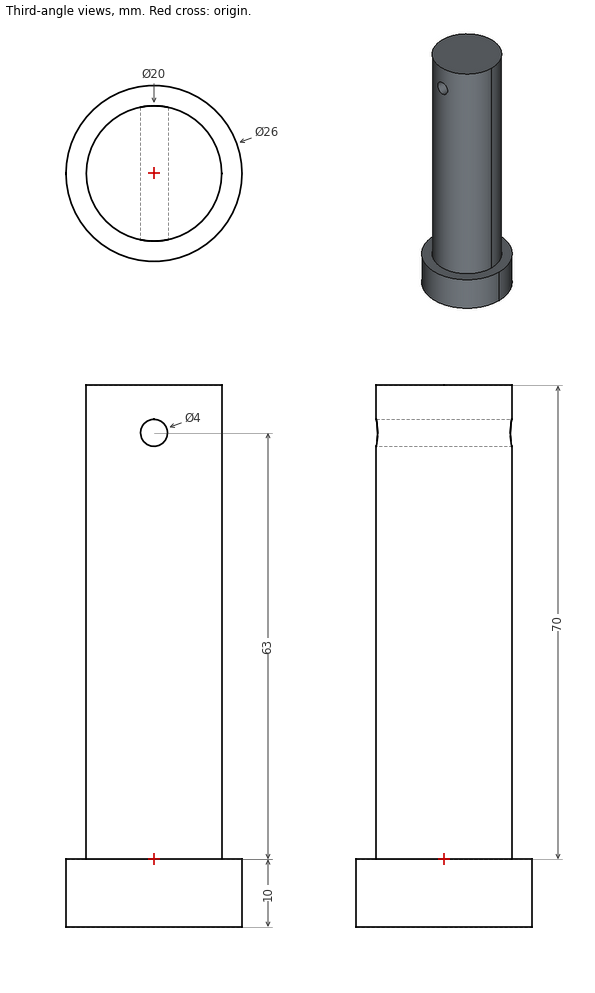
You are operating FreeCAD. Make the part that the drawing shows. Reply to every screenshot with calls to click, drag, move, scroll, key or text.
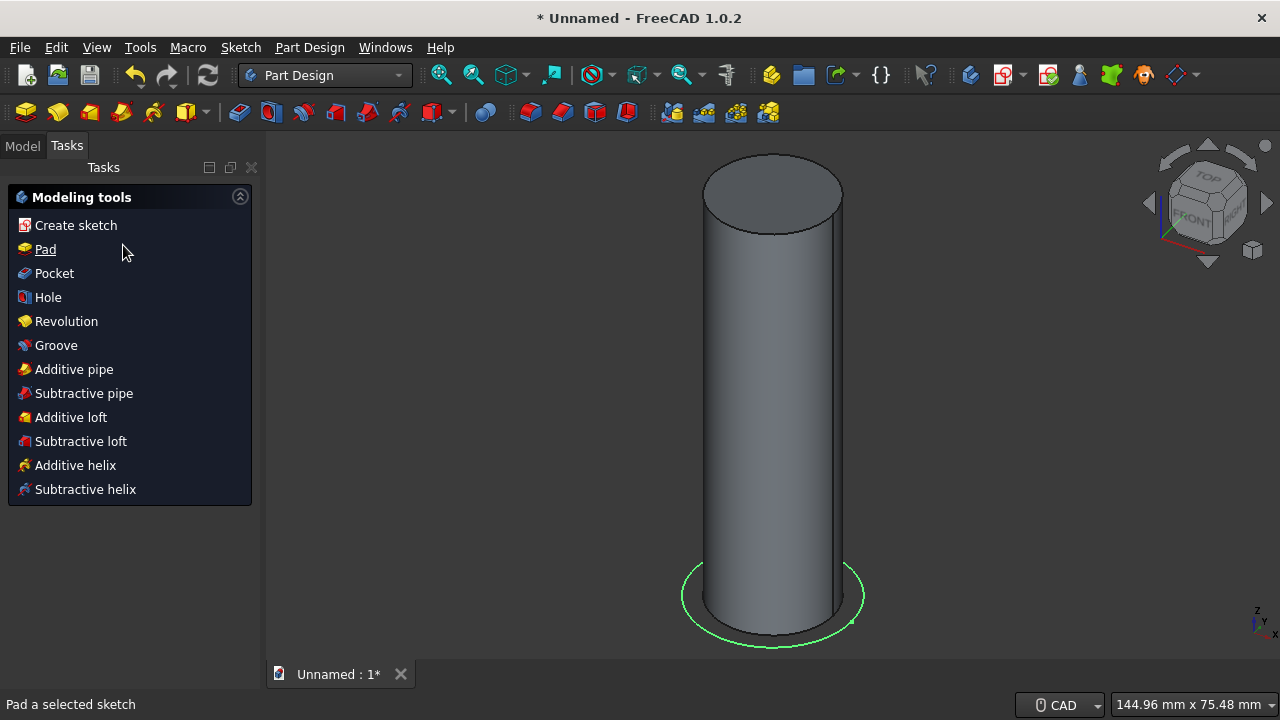
click(26, 112)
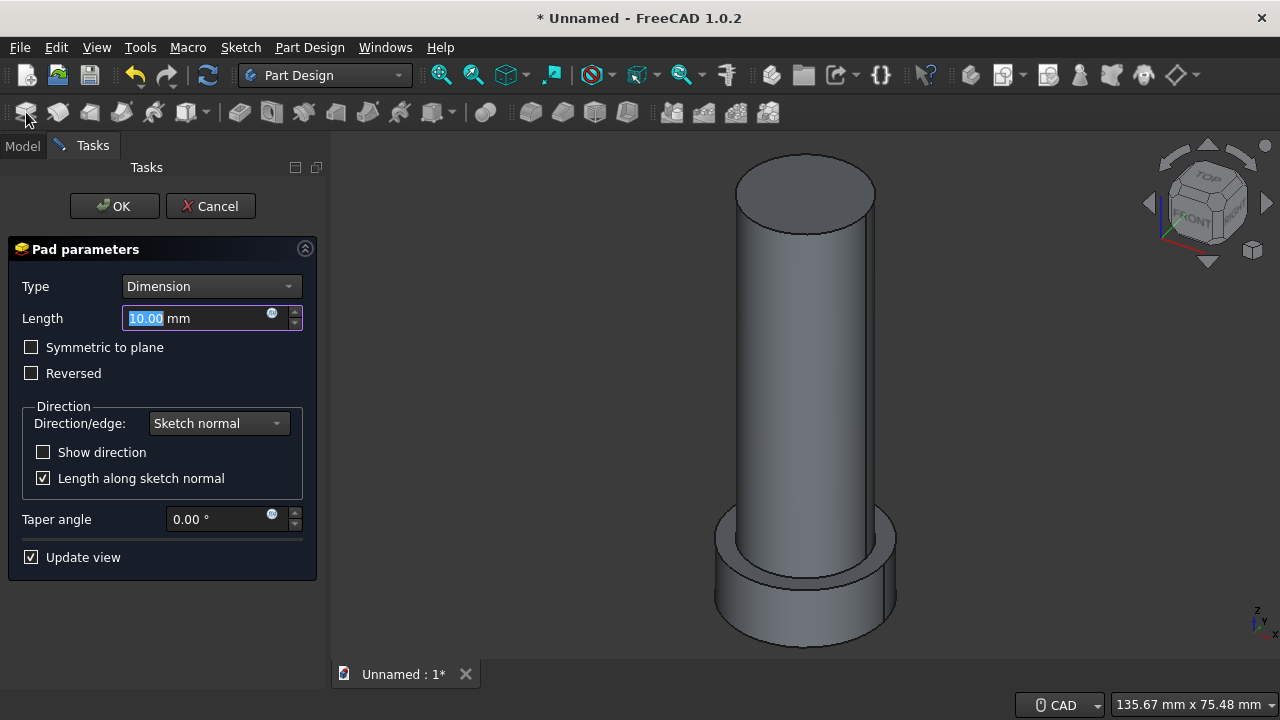
text(10)
key(Tab)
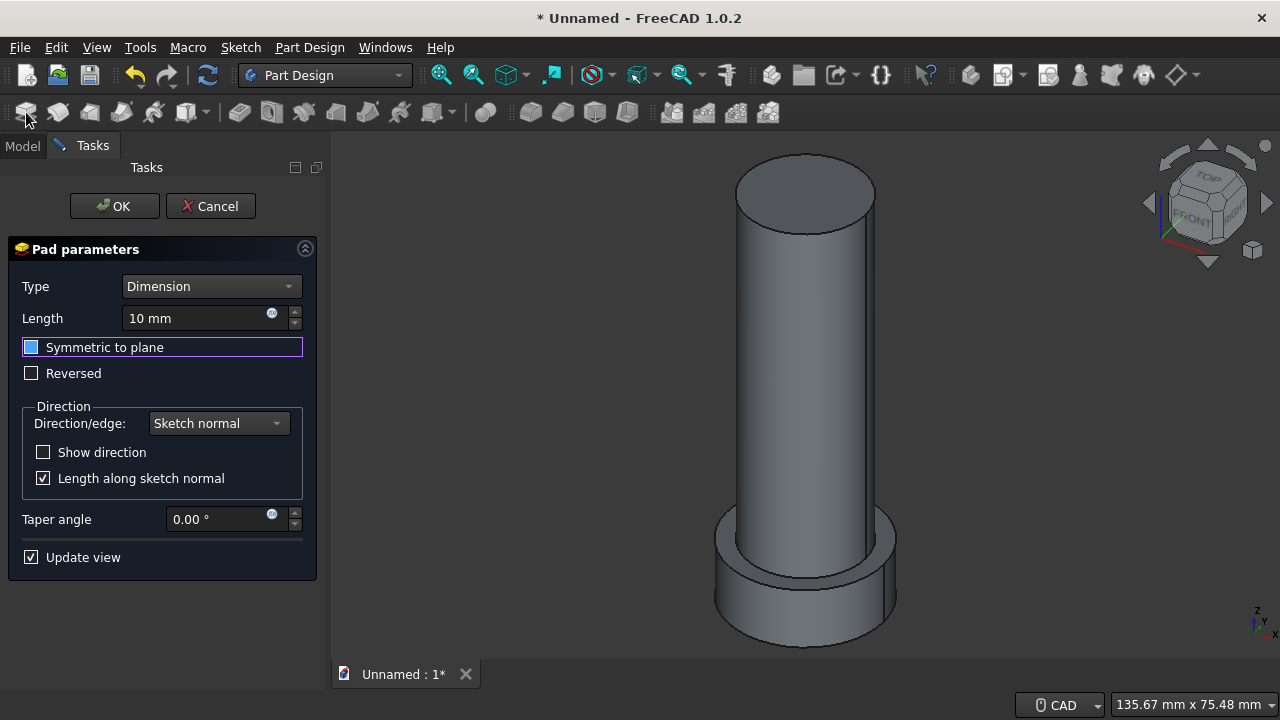
click(30, 373)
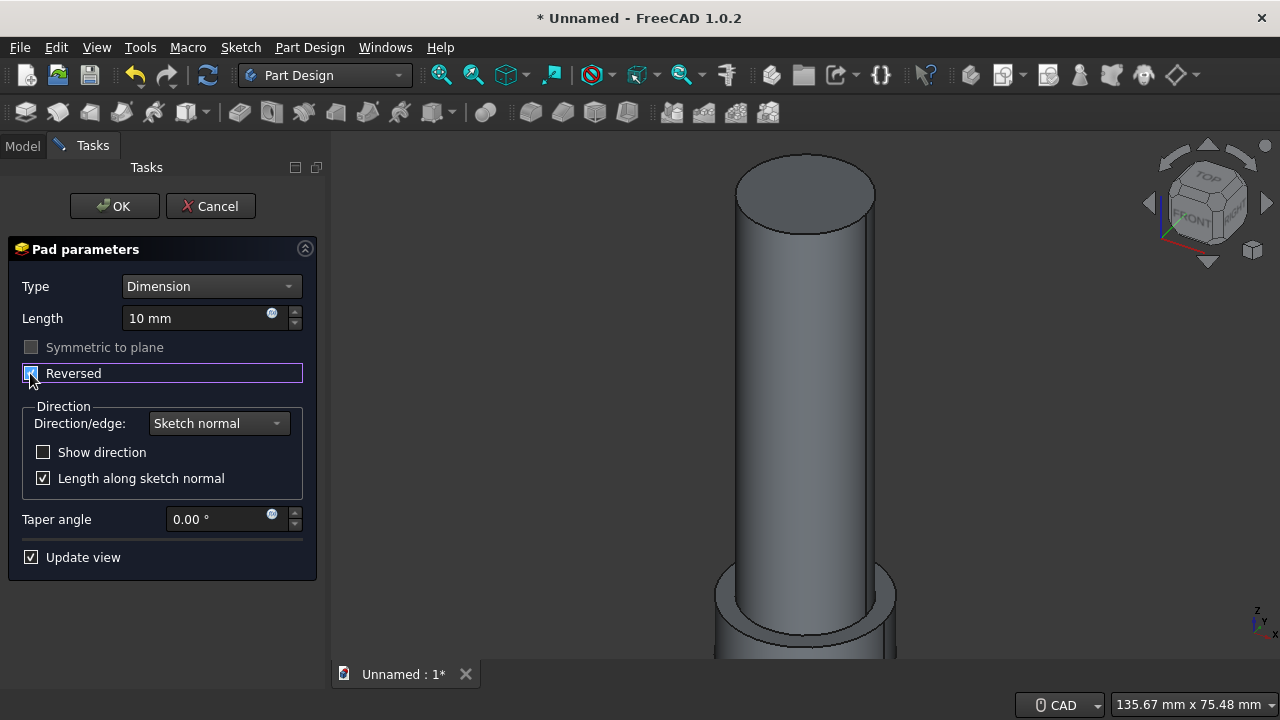
click(115, 206)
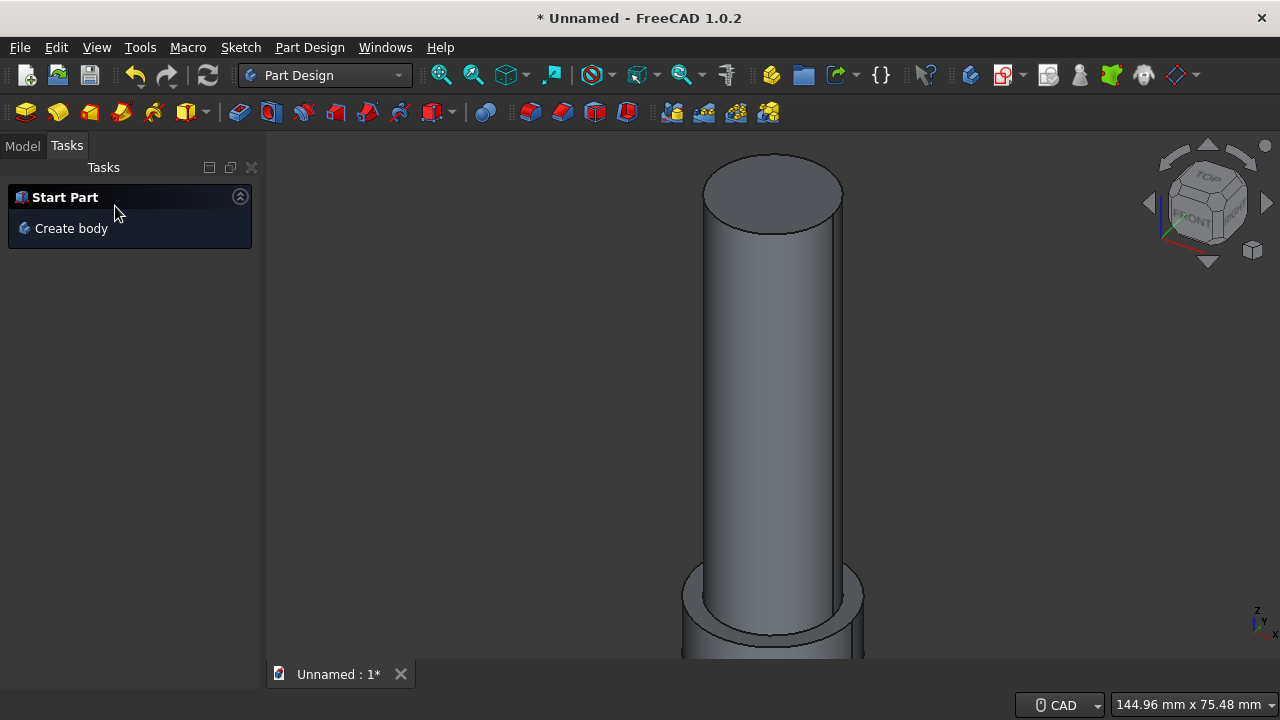
click(442, 76)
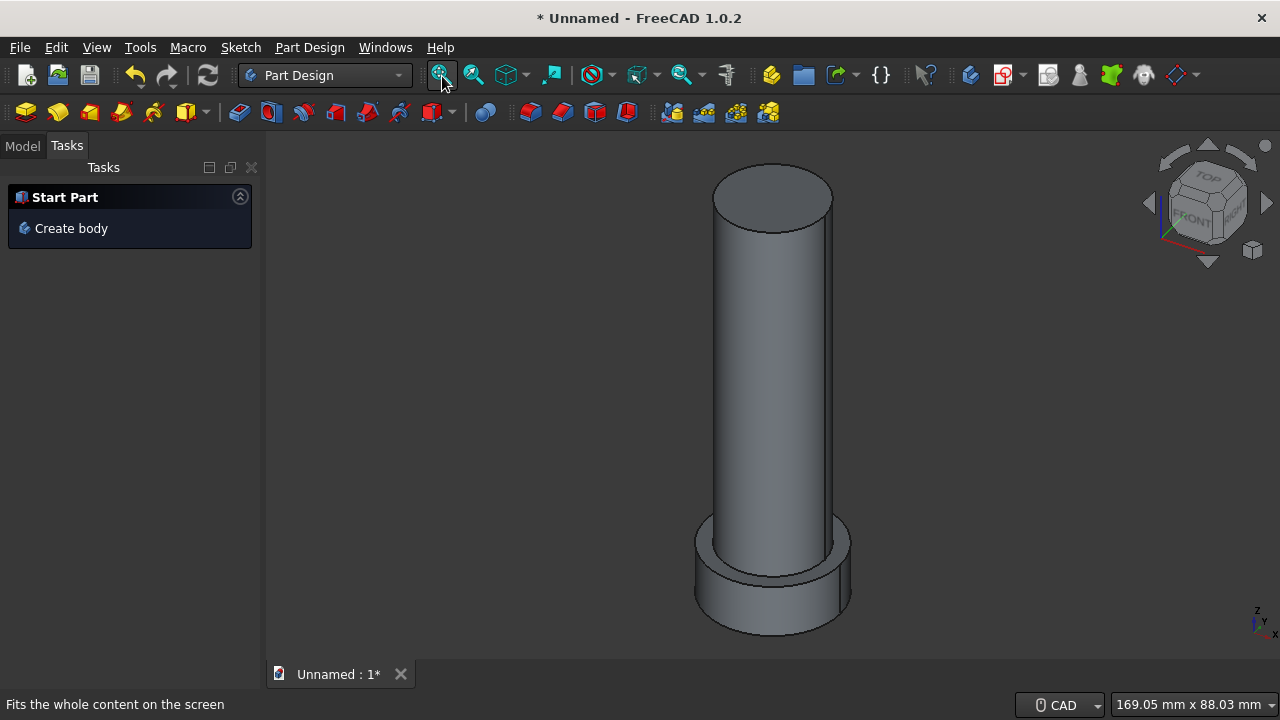
click(1004, 76)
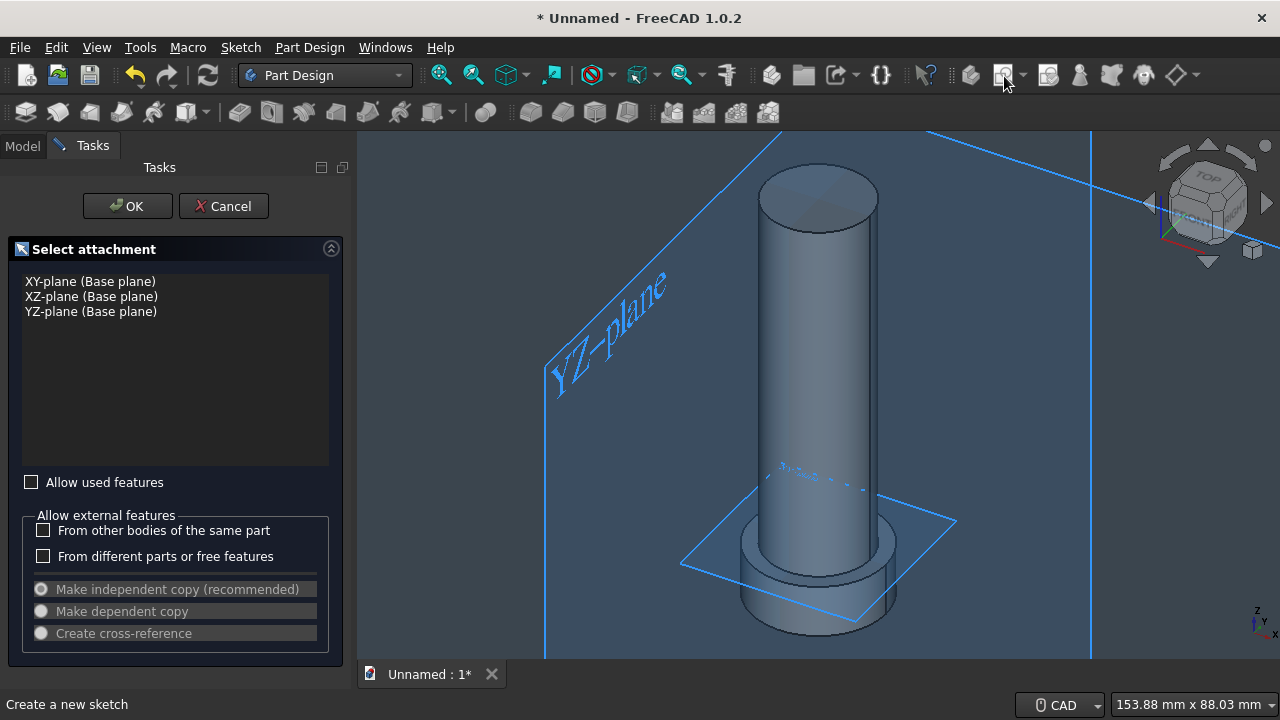
click(82, 296)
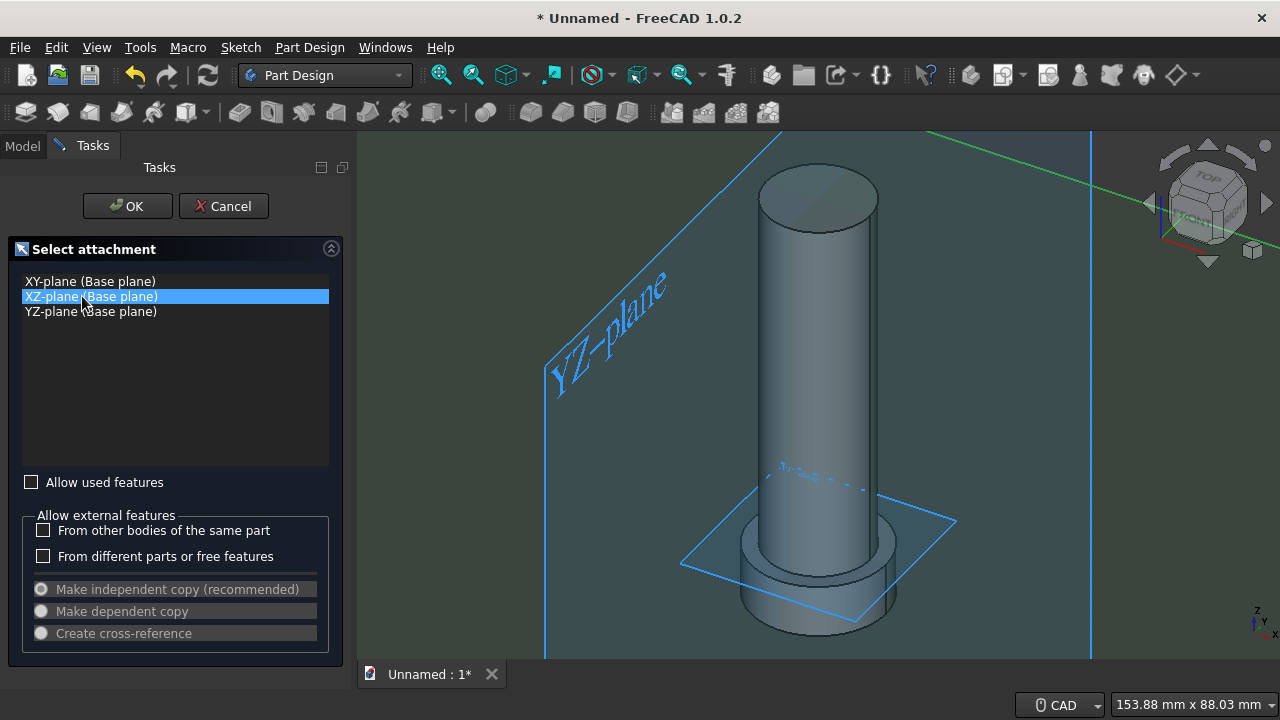
click(128, 206)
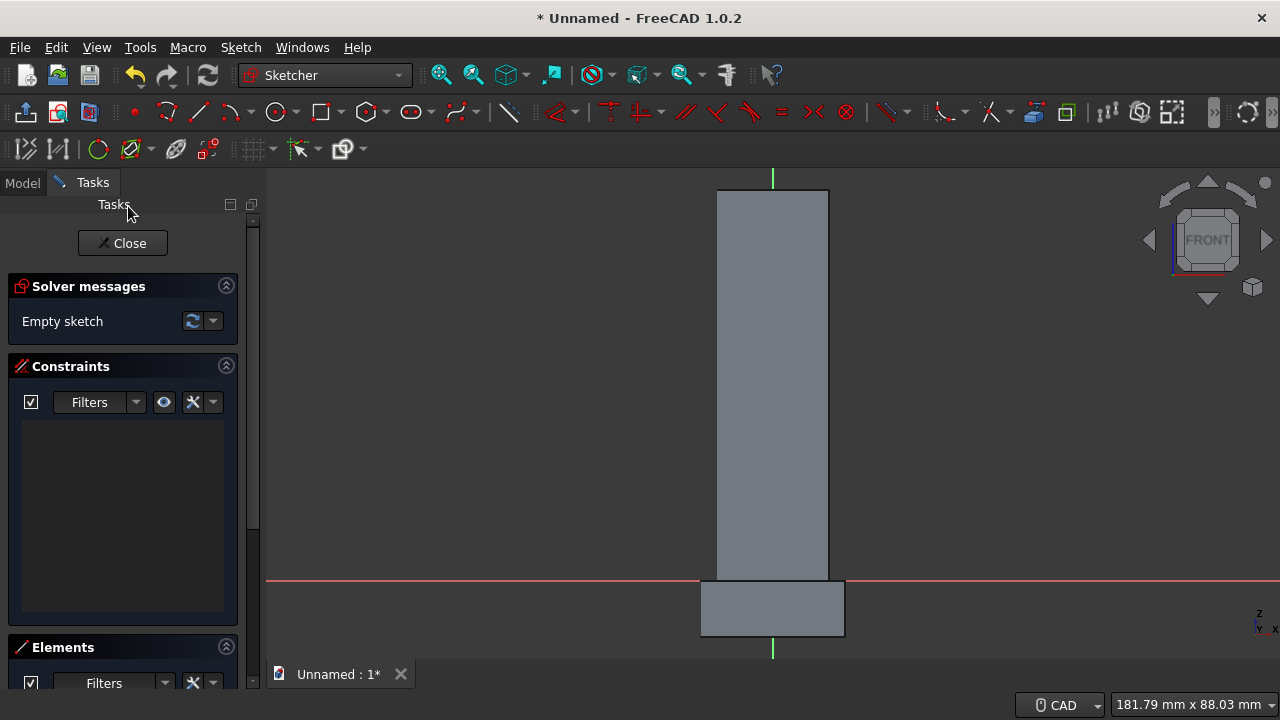
click(90, 112)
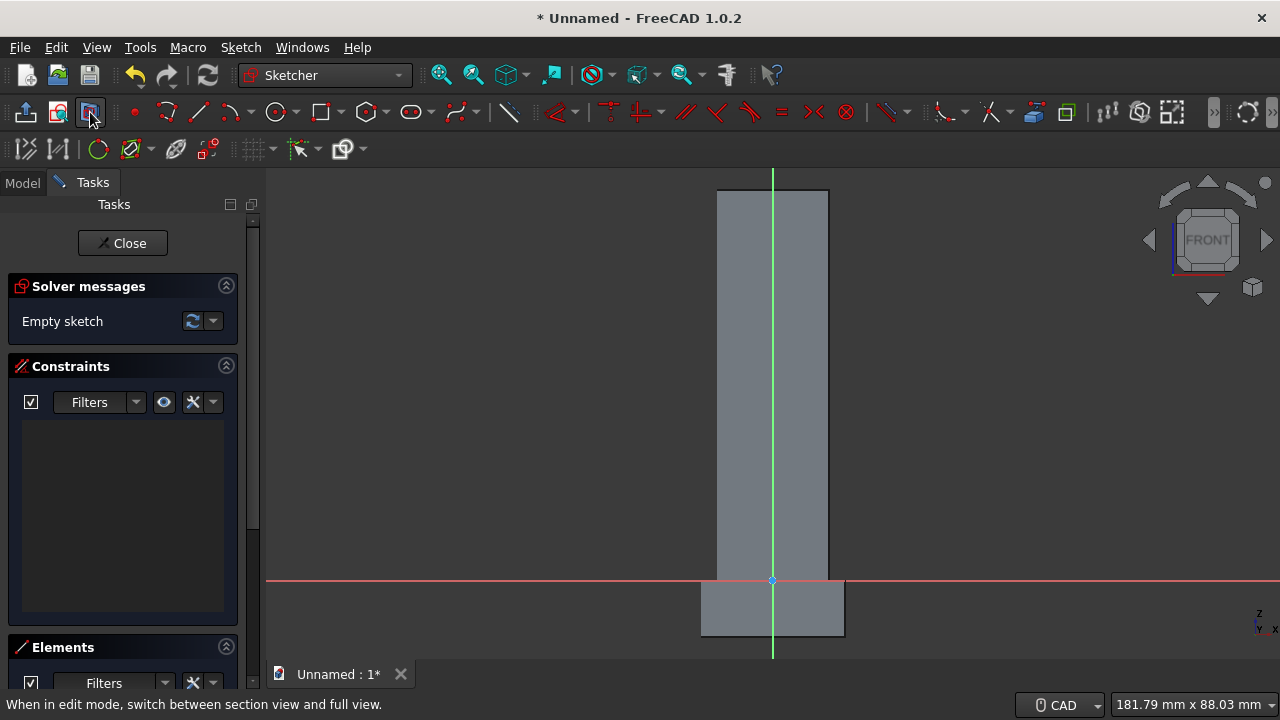
scroll(778, 215, up, 13)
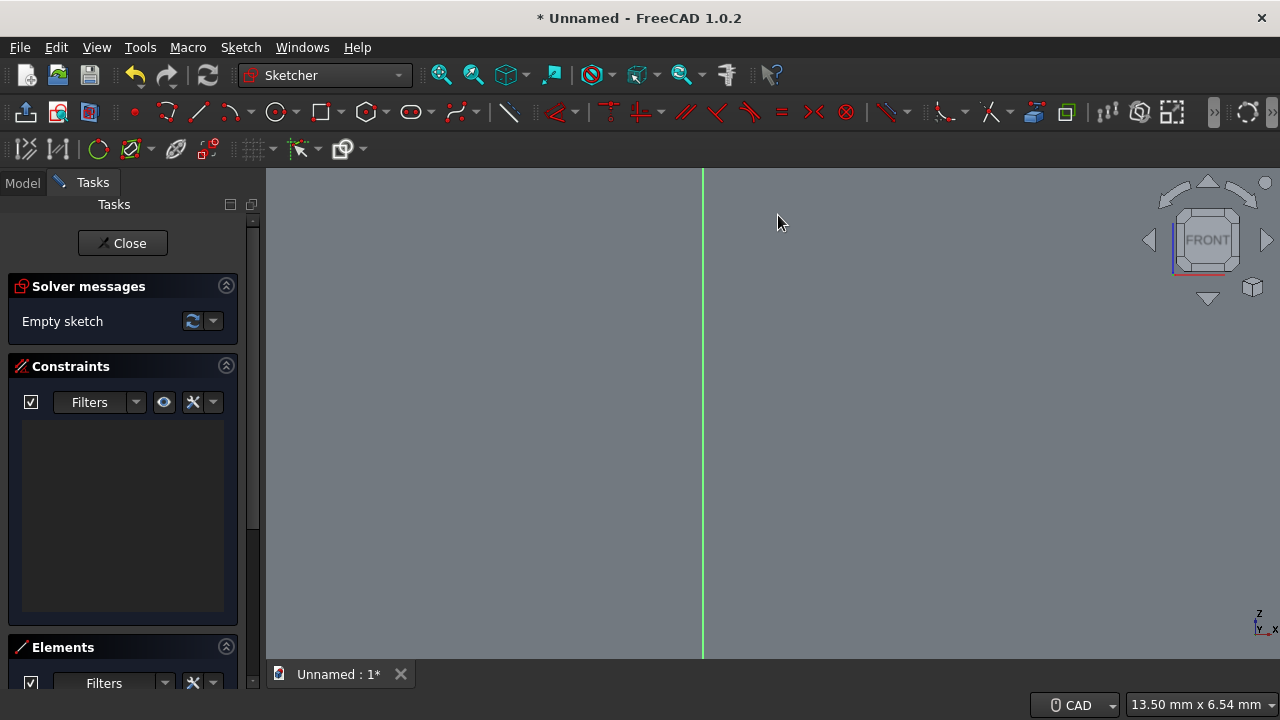
click(276, 112)